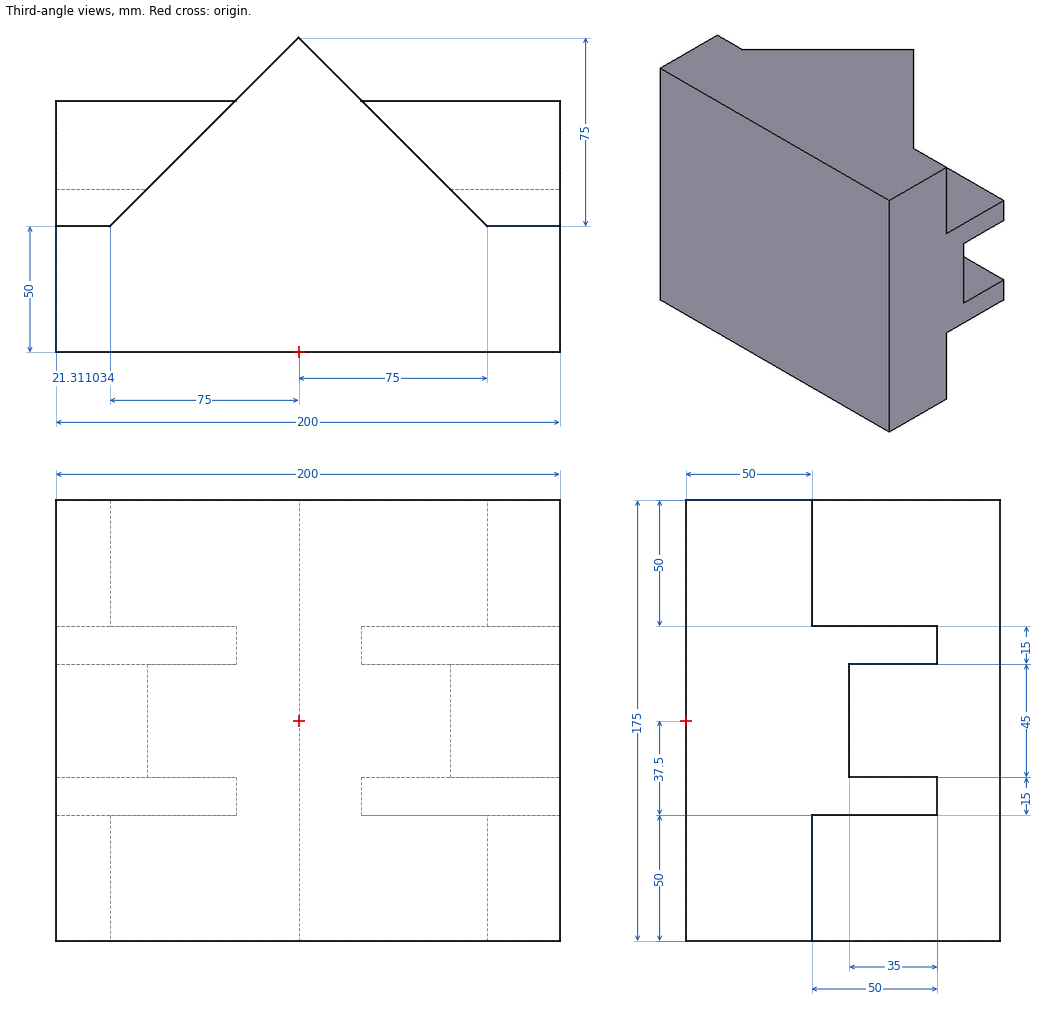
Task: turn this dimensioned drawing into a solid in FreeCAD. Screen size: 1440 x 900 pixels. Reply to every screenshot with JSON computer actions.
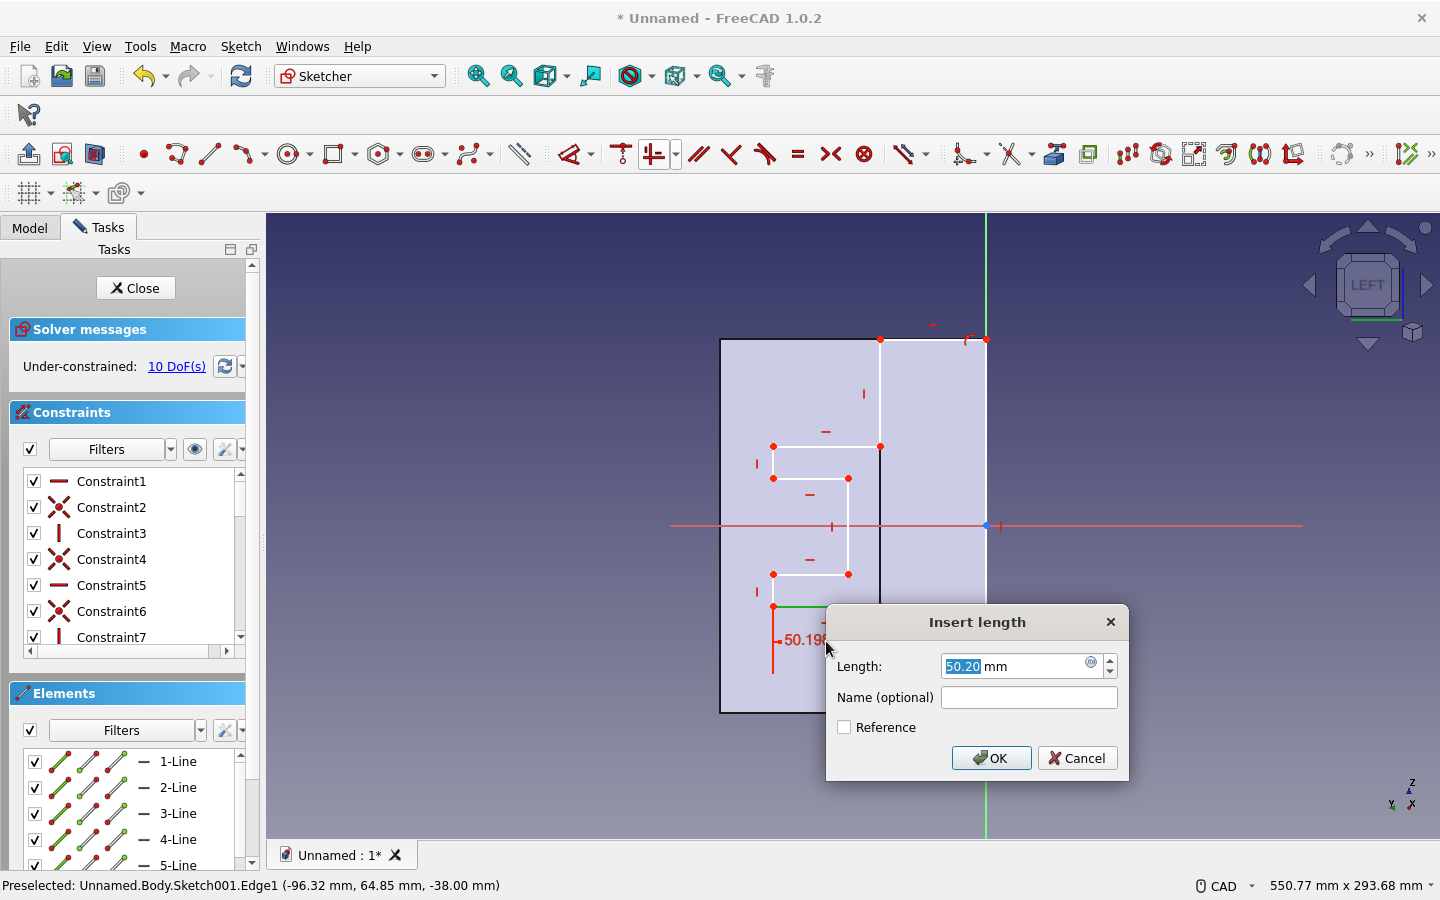
{"action": "type", "text": "50"}
{"action": "key", "text": "Return"}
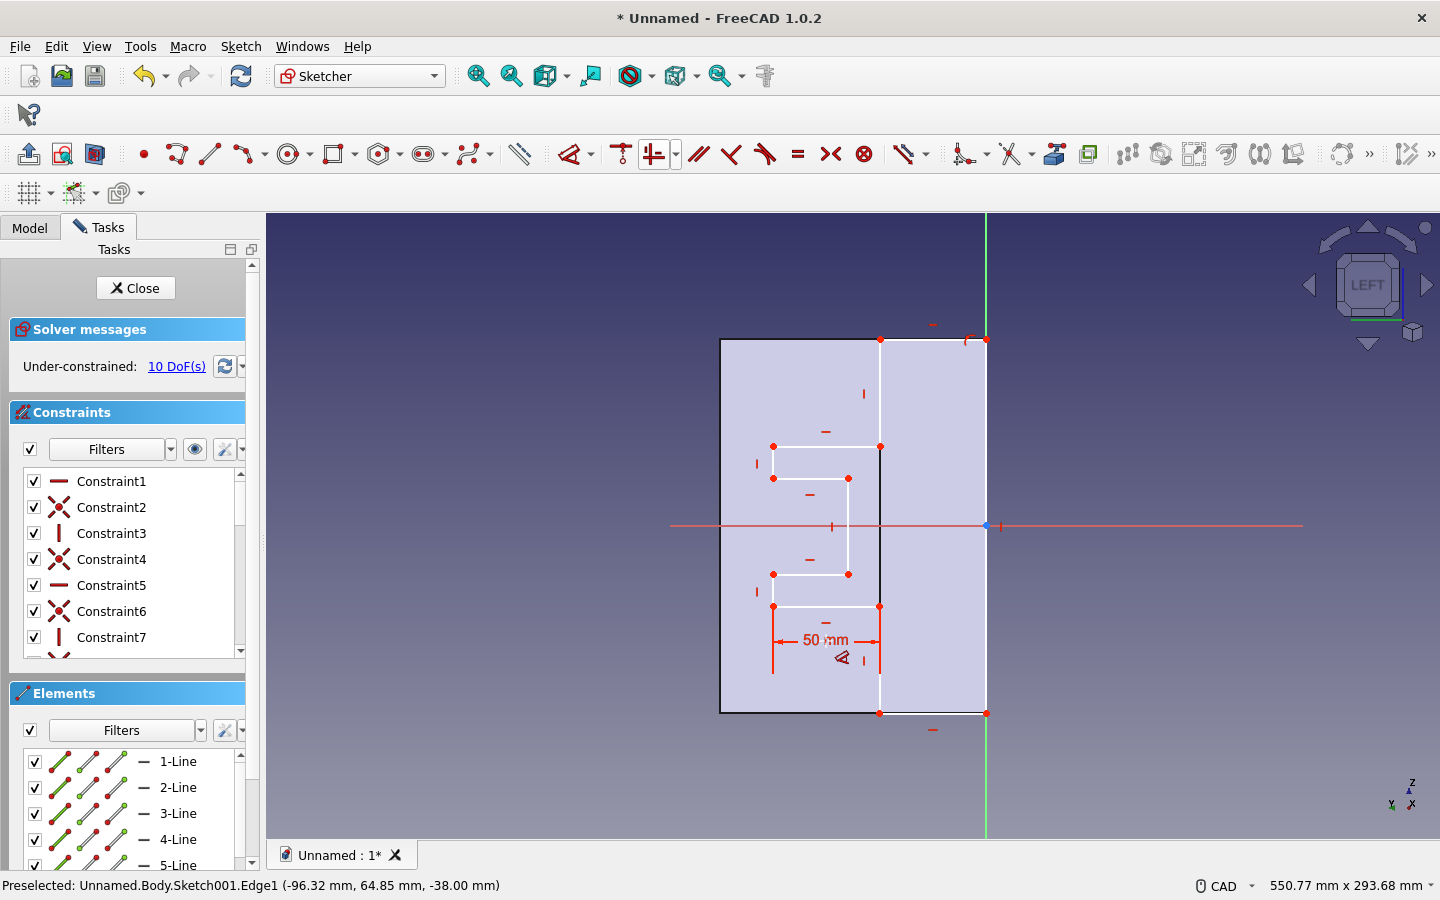
{"action": "scroll", "coordinate": [773, 597], "scroll_direction": "up", "scroll_amount": 2}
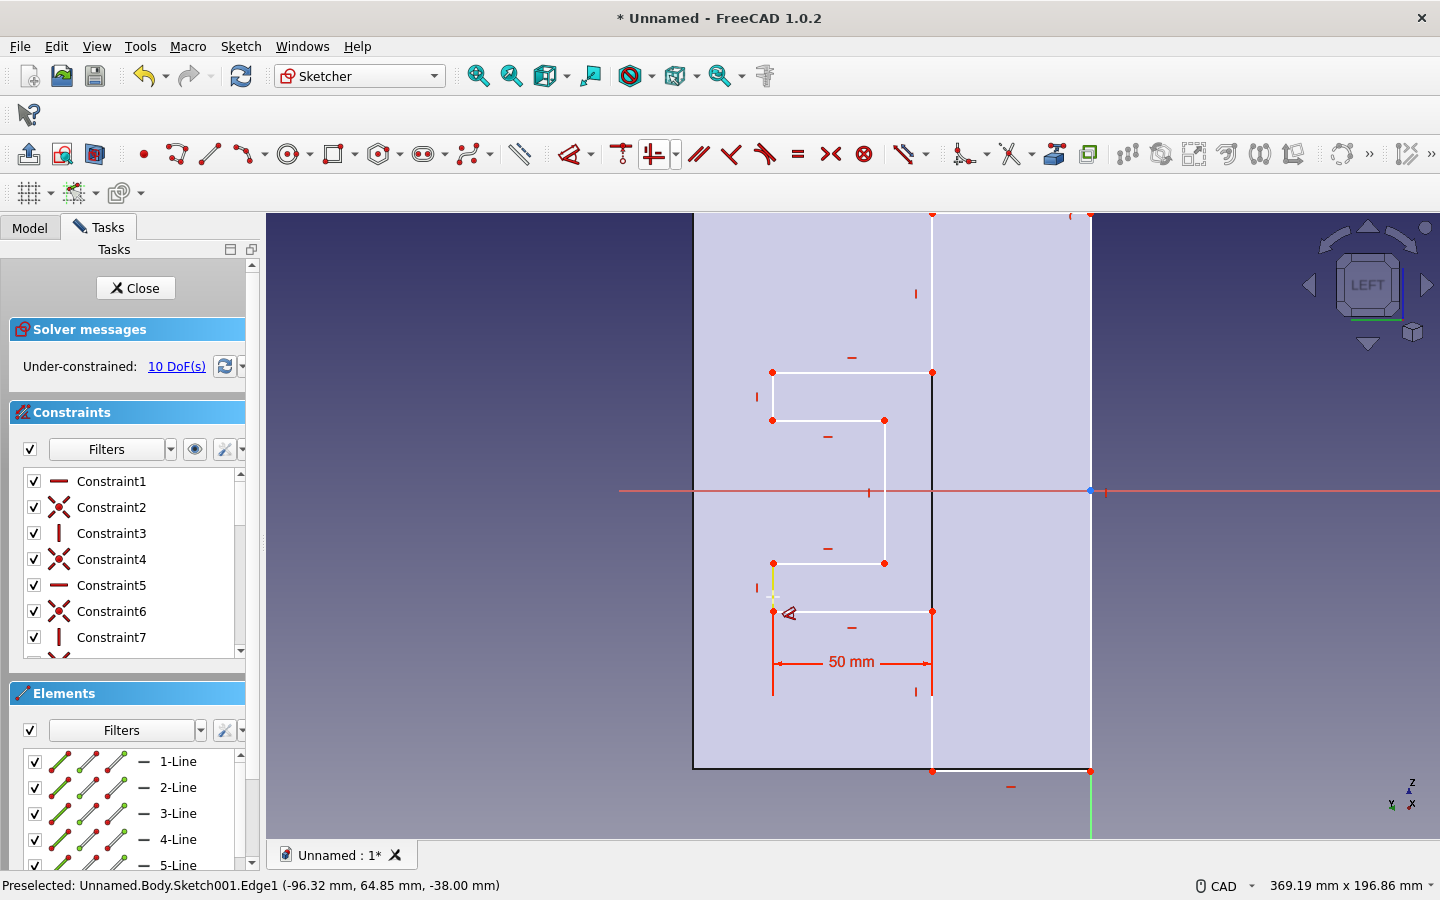
{"action": "left_click", "coordinate": [773, 597]}
{"action": "left_click", "coordinate": [739, 588]}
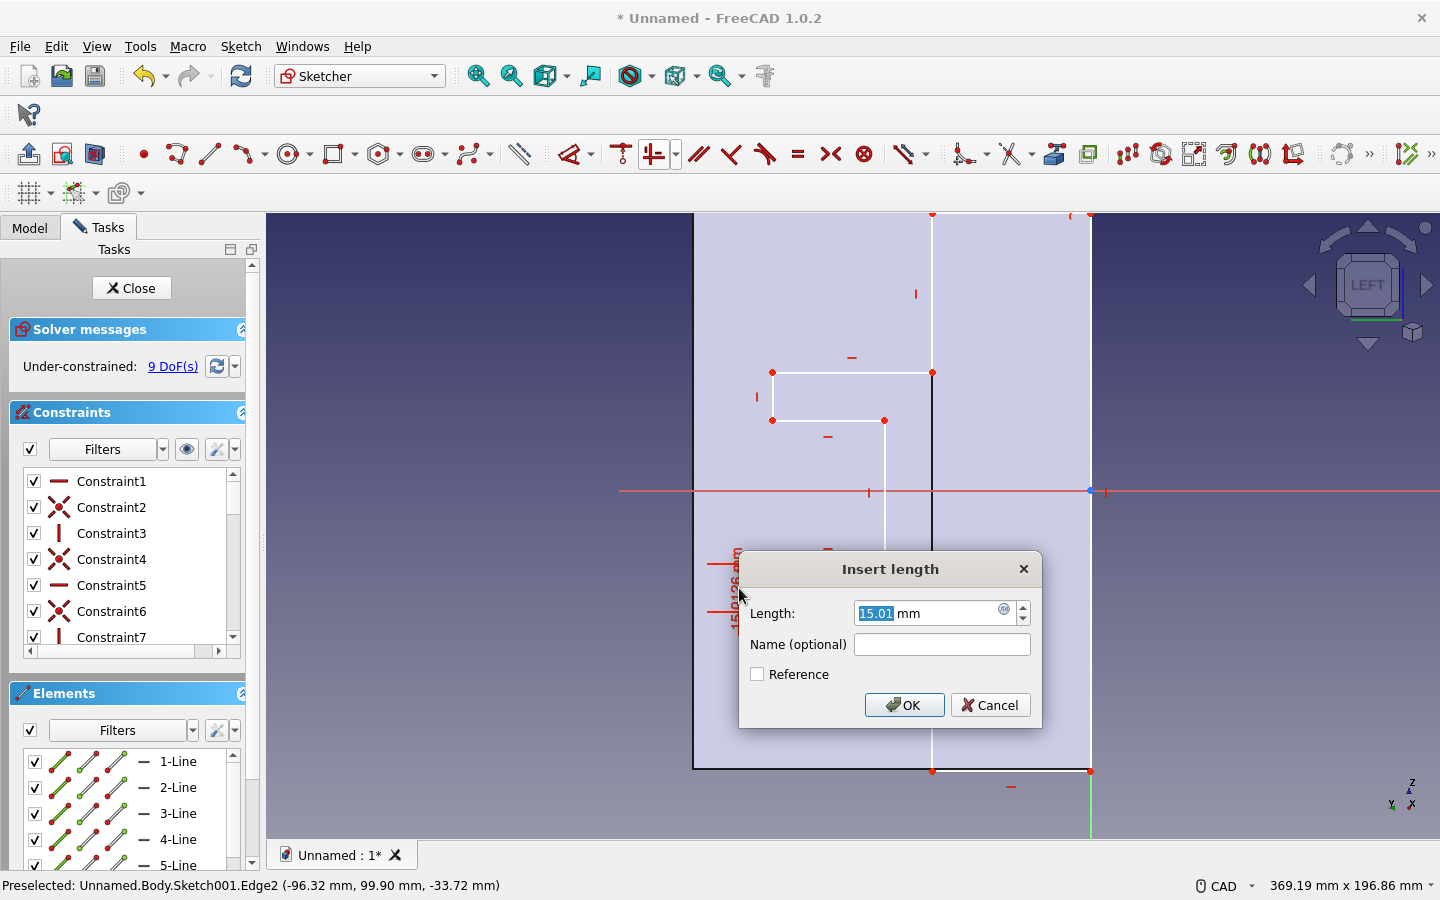
{"action": "type", "text": "15"}
{"action": "key", "text": "Return"}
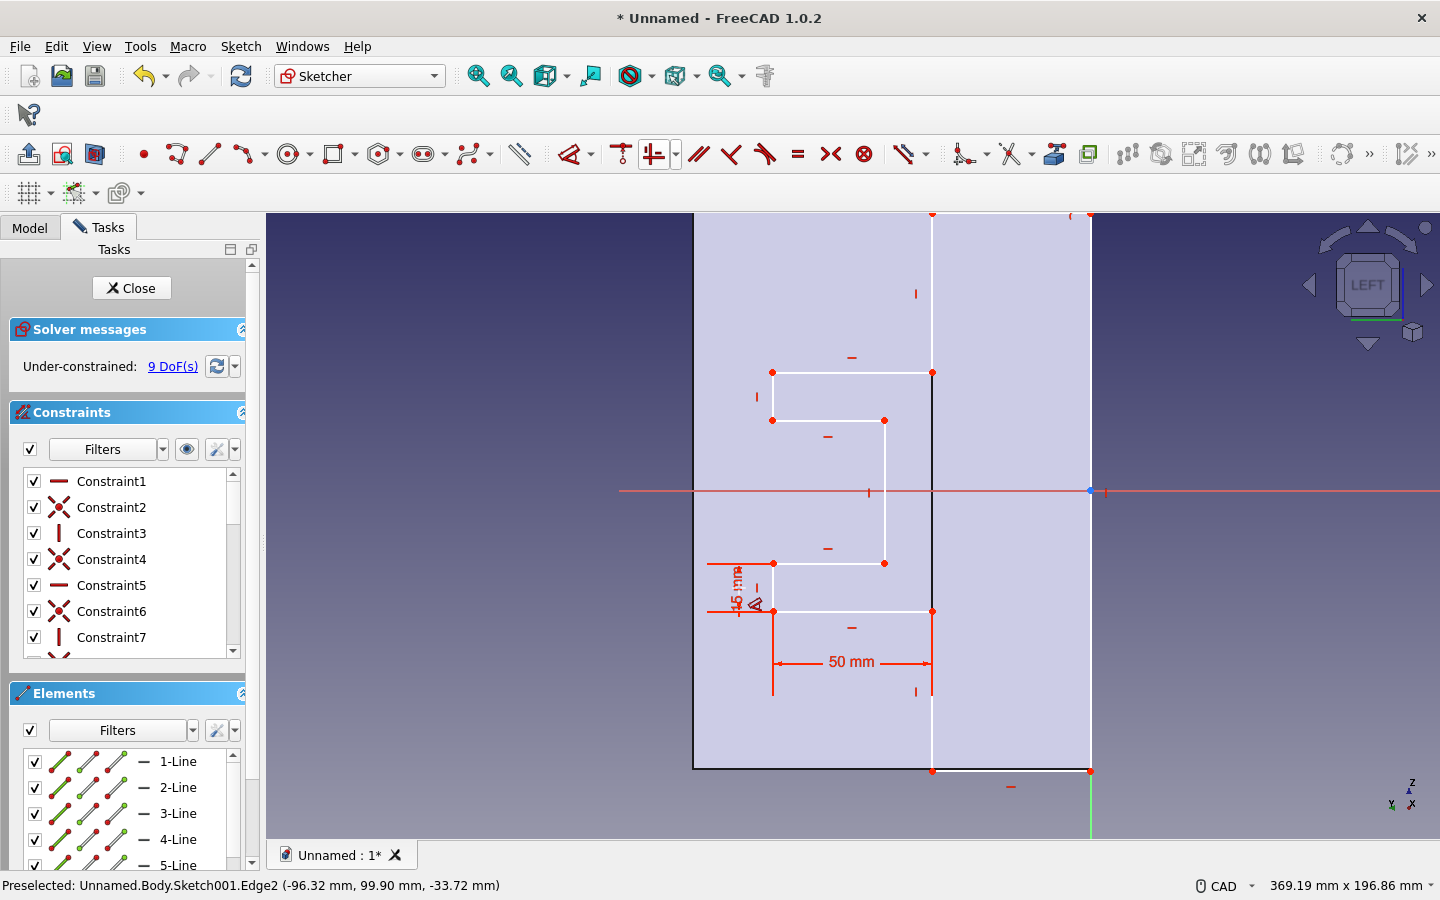
{"action": "left_click", "coordinate": [807, 564]}
{"action": "left_click", "coordinate": [829, 598]}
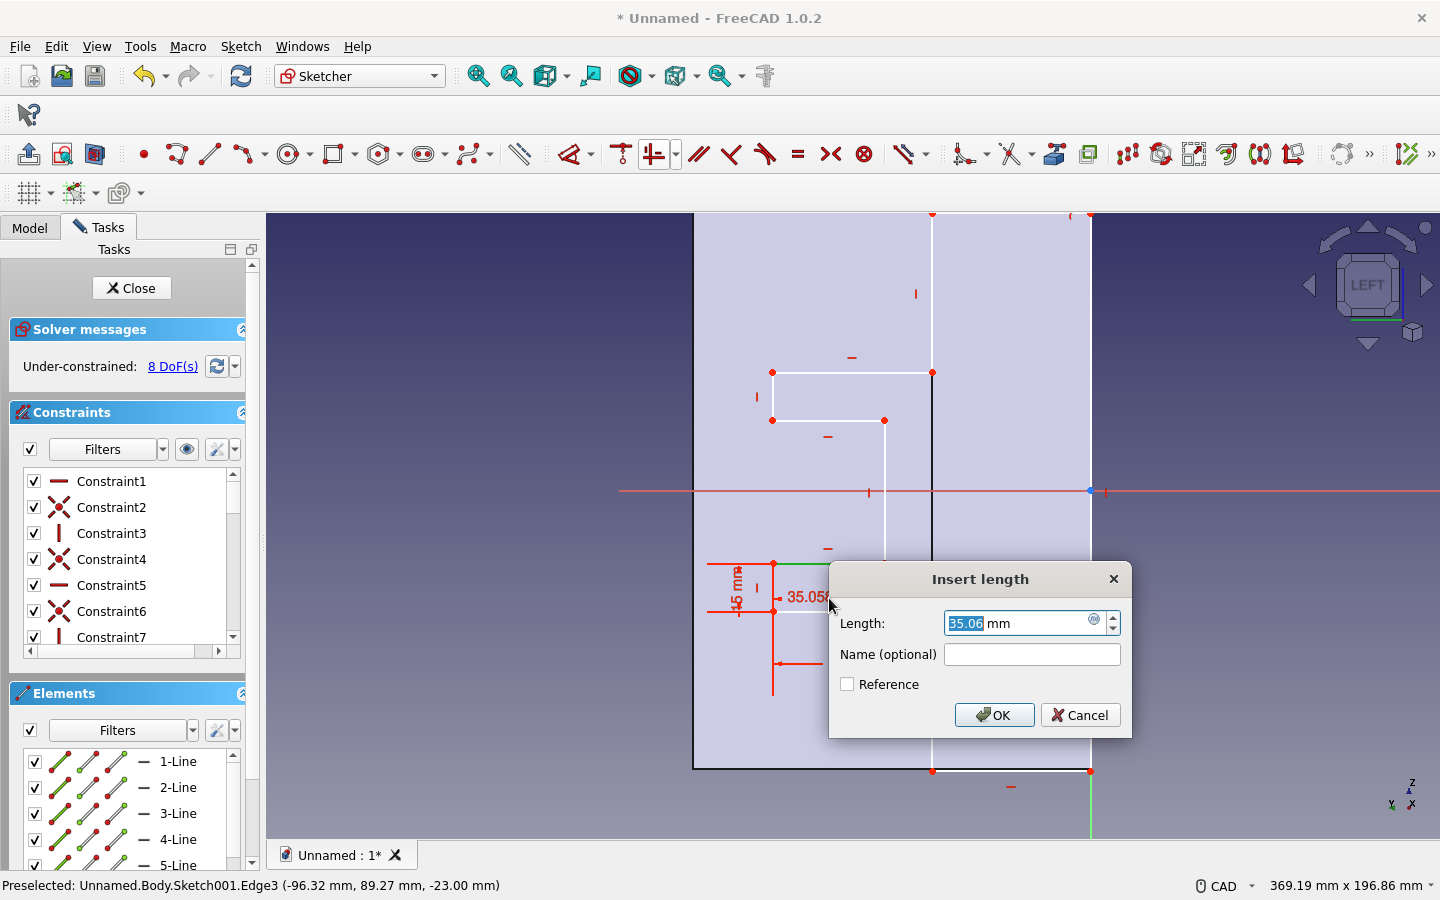
{"action": "type", "text": "35"}
{"action": "key", "text": "Return"}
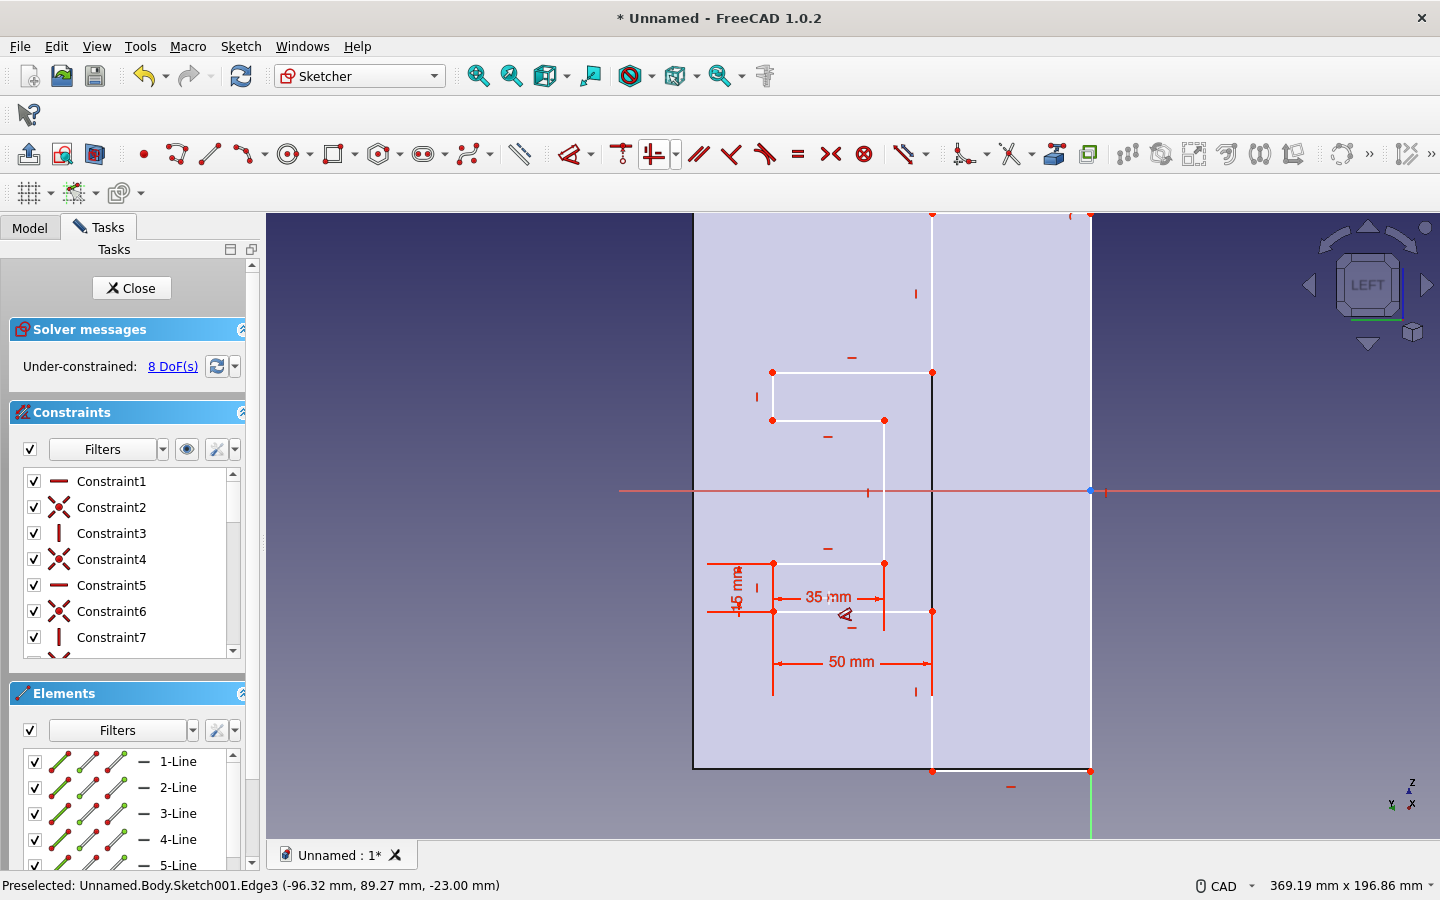
{"action": "left_click", "coordinate": [884, 521]}
{"action": "left_click", "coordinate": [850, 459]}